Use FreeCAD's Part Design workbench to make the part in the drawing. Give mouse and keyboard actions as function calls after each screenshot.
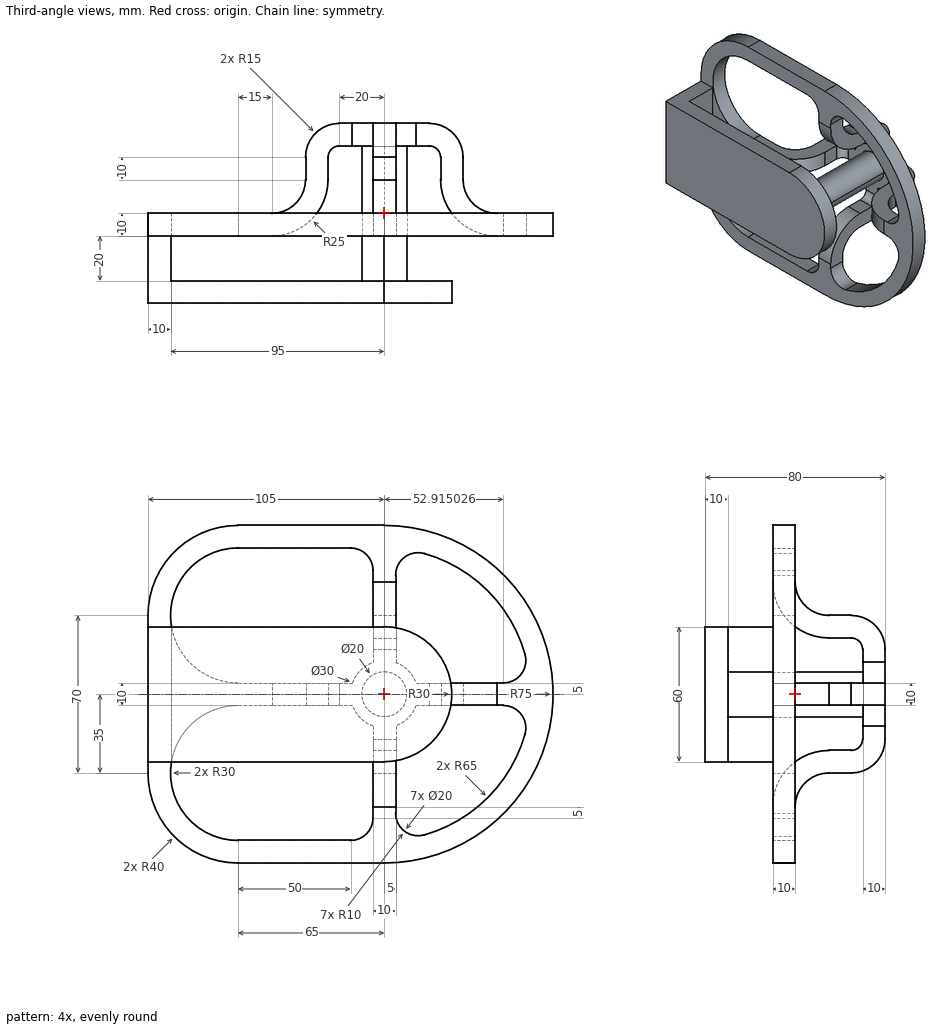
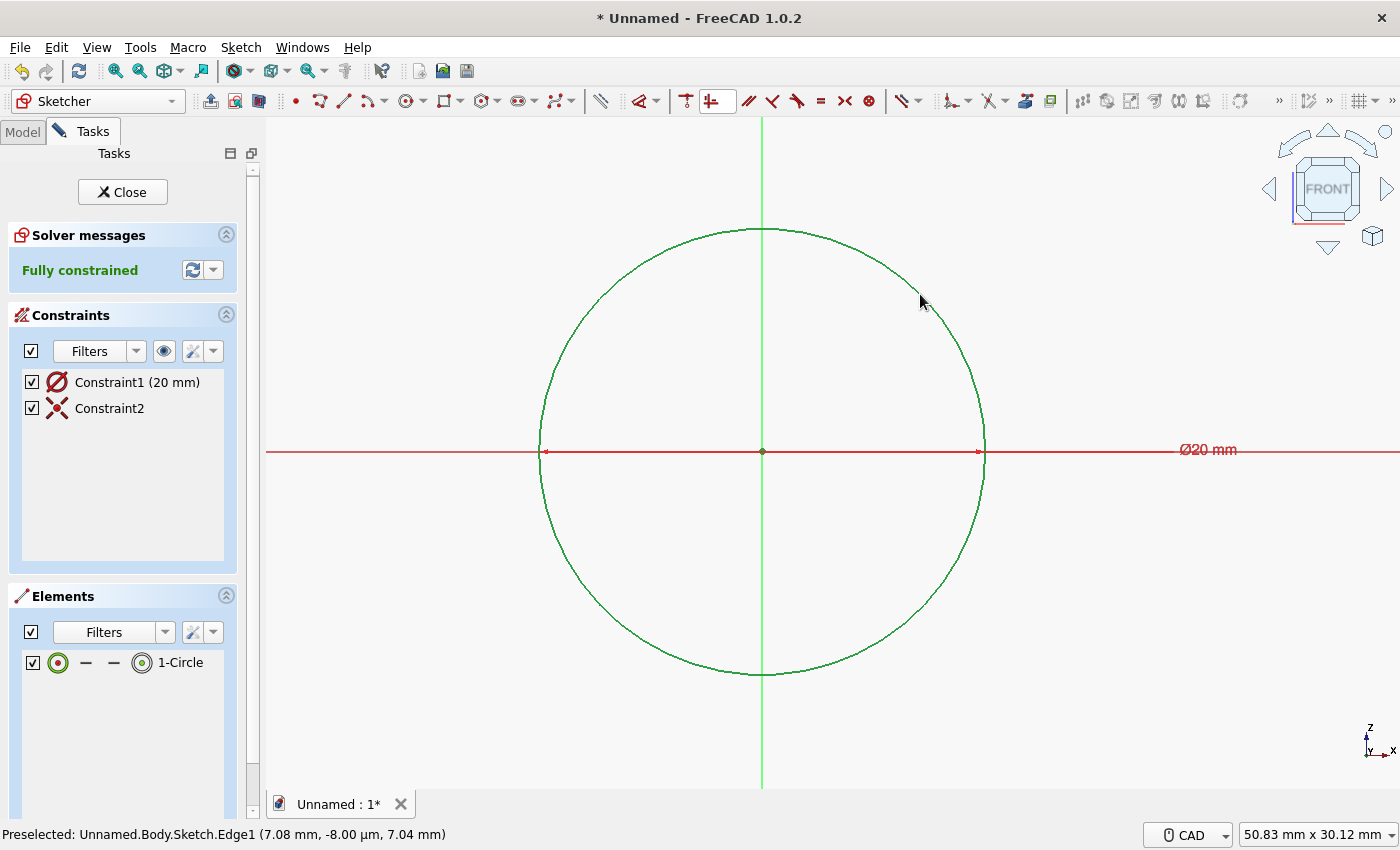
click(123, 192)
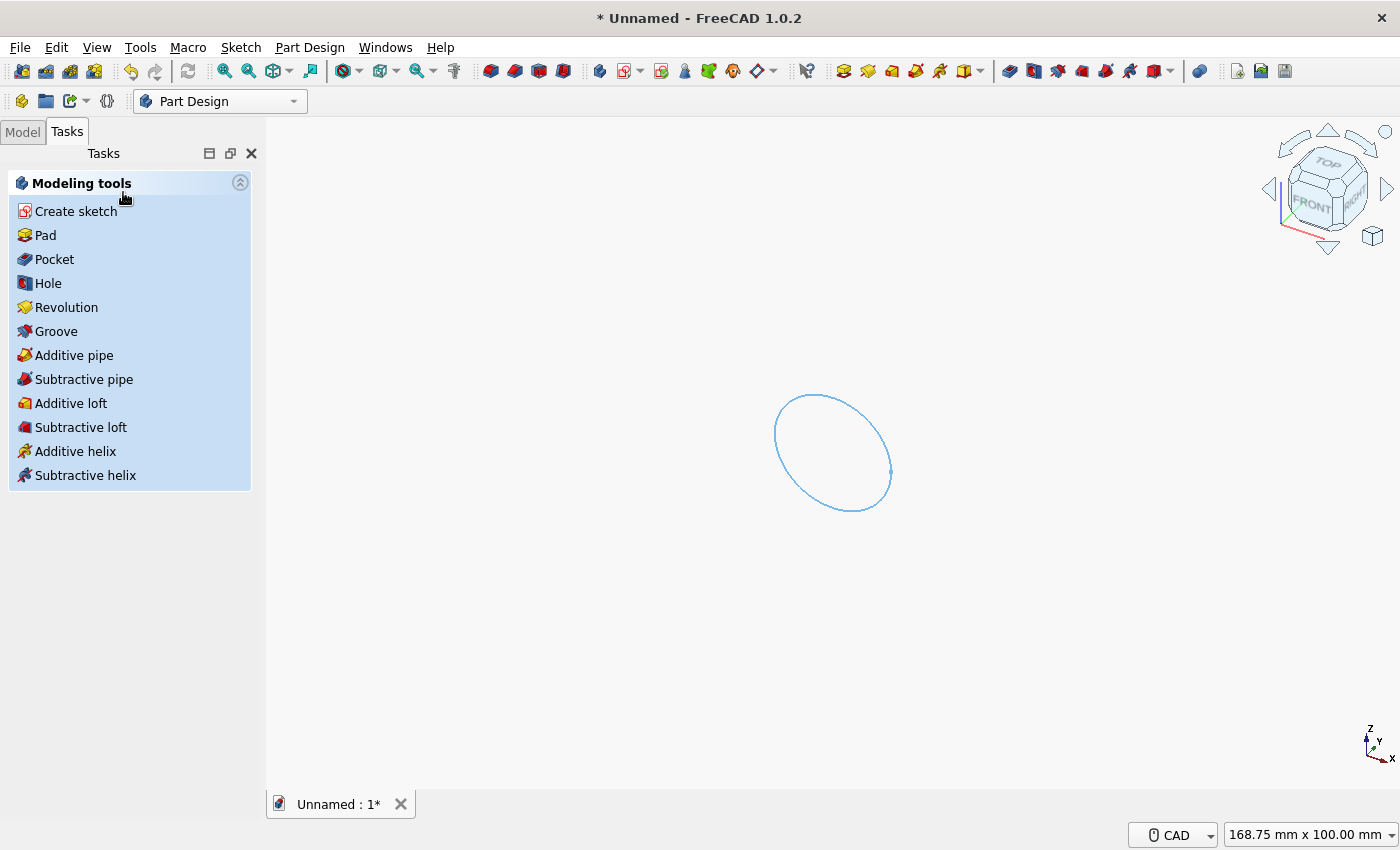
click(844, 72)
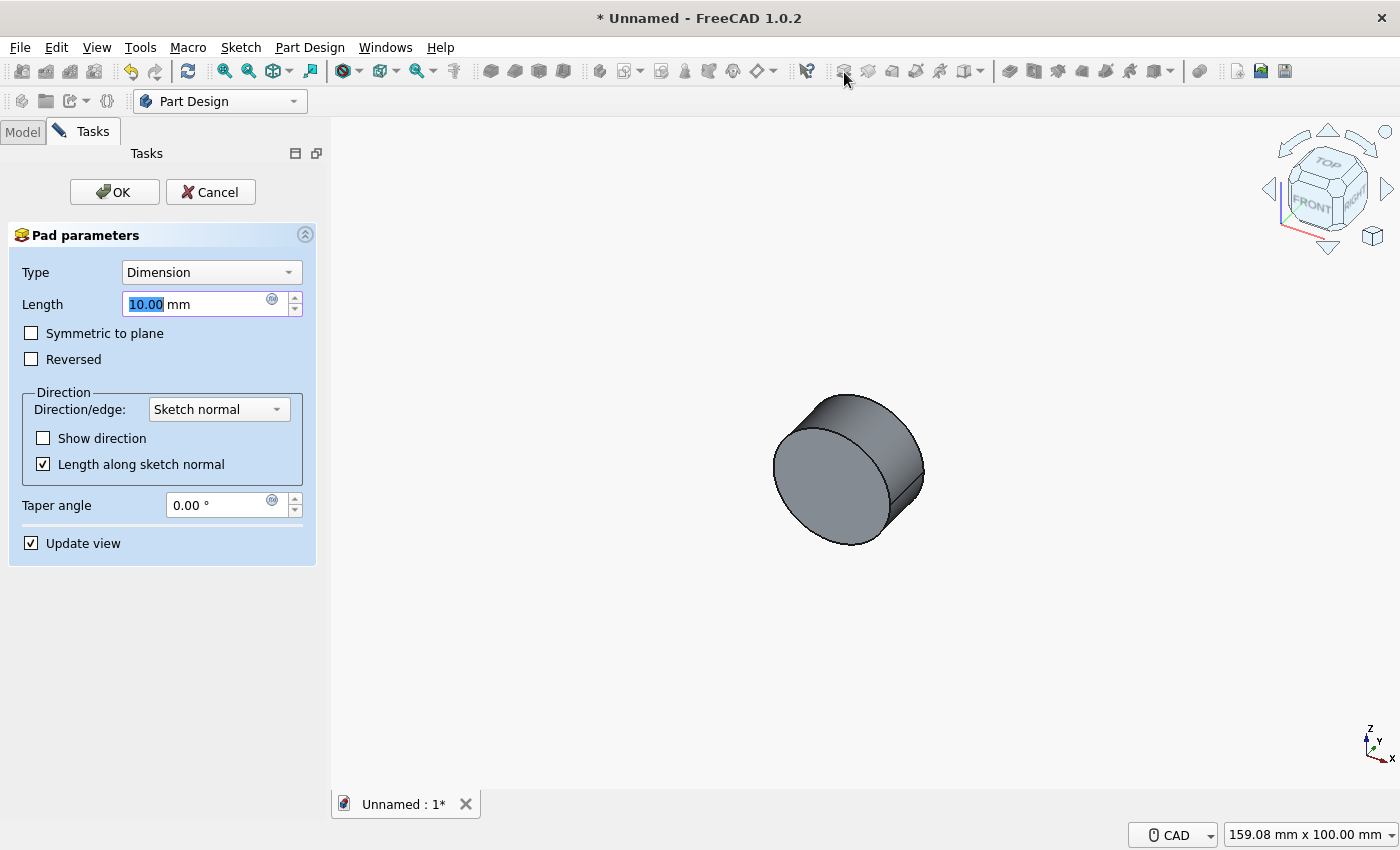
text(80)
key(Tab)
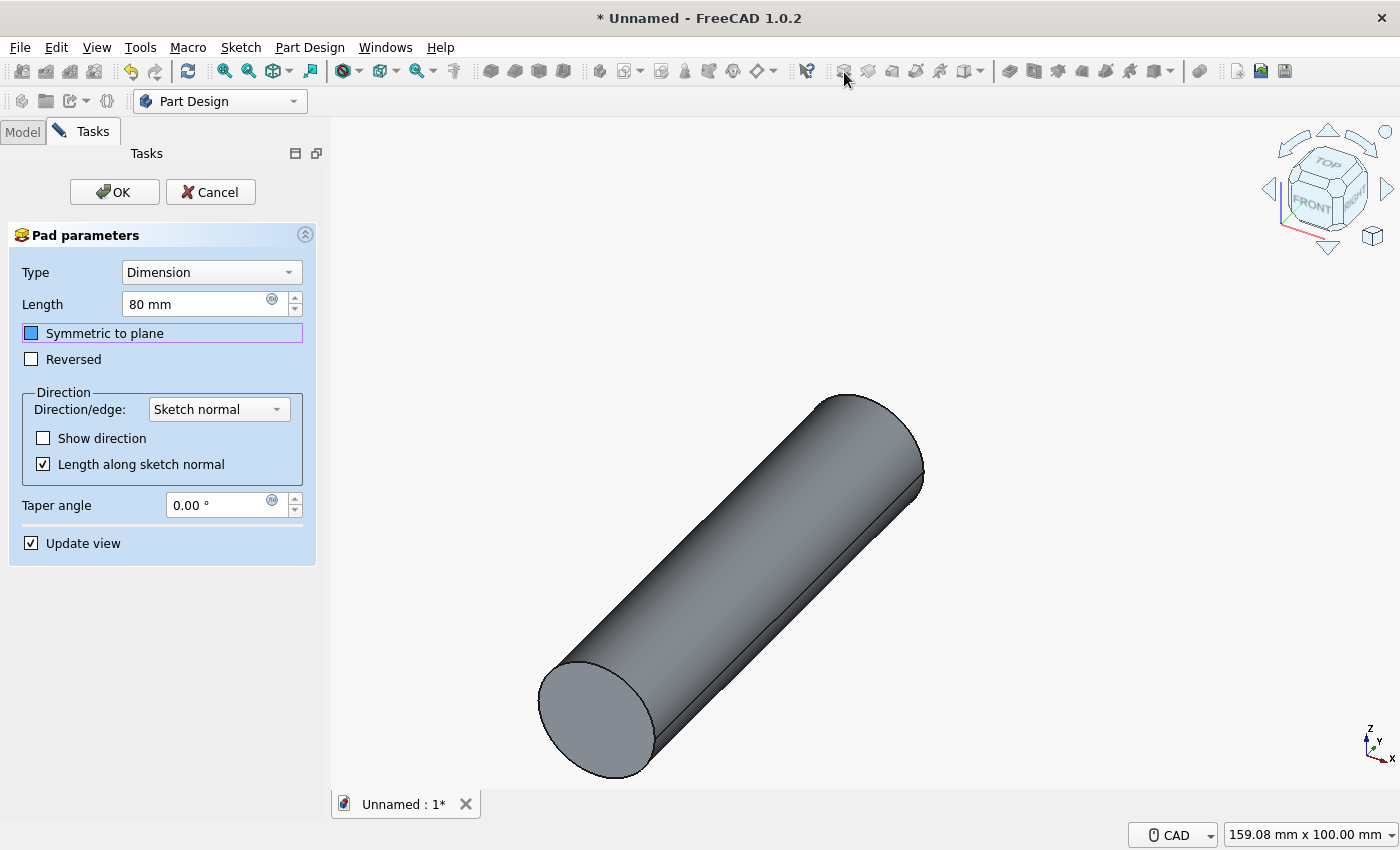
click(30, 333)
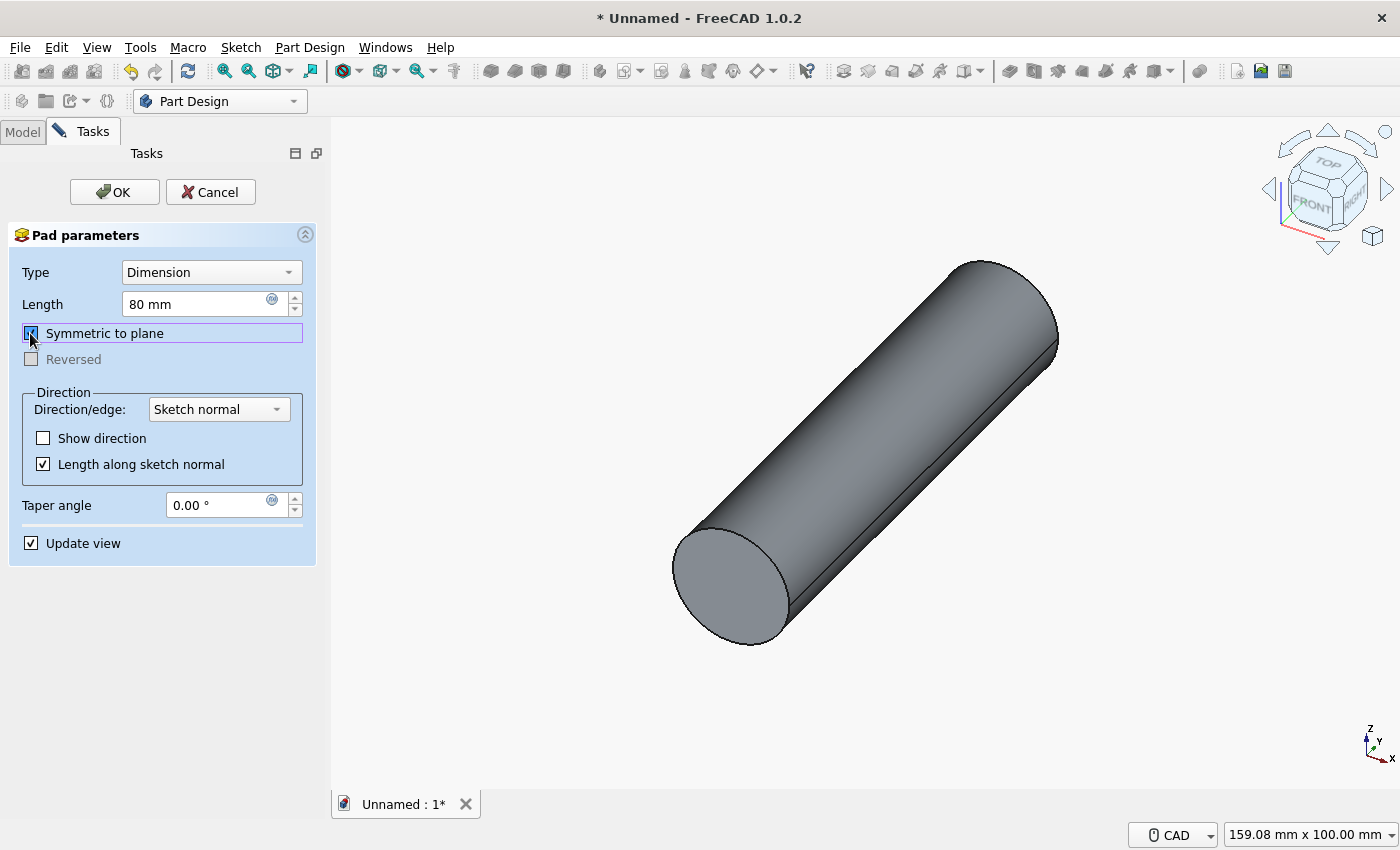
click(115, 192)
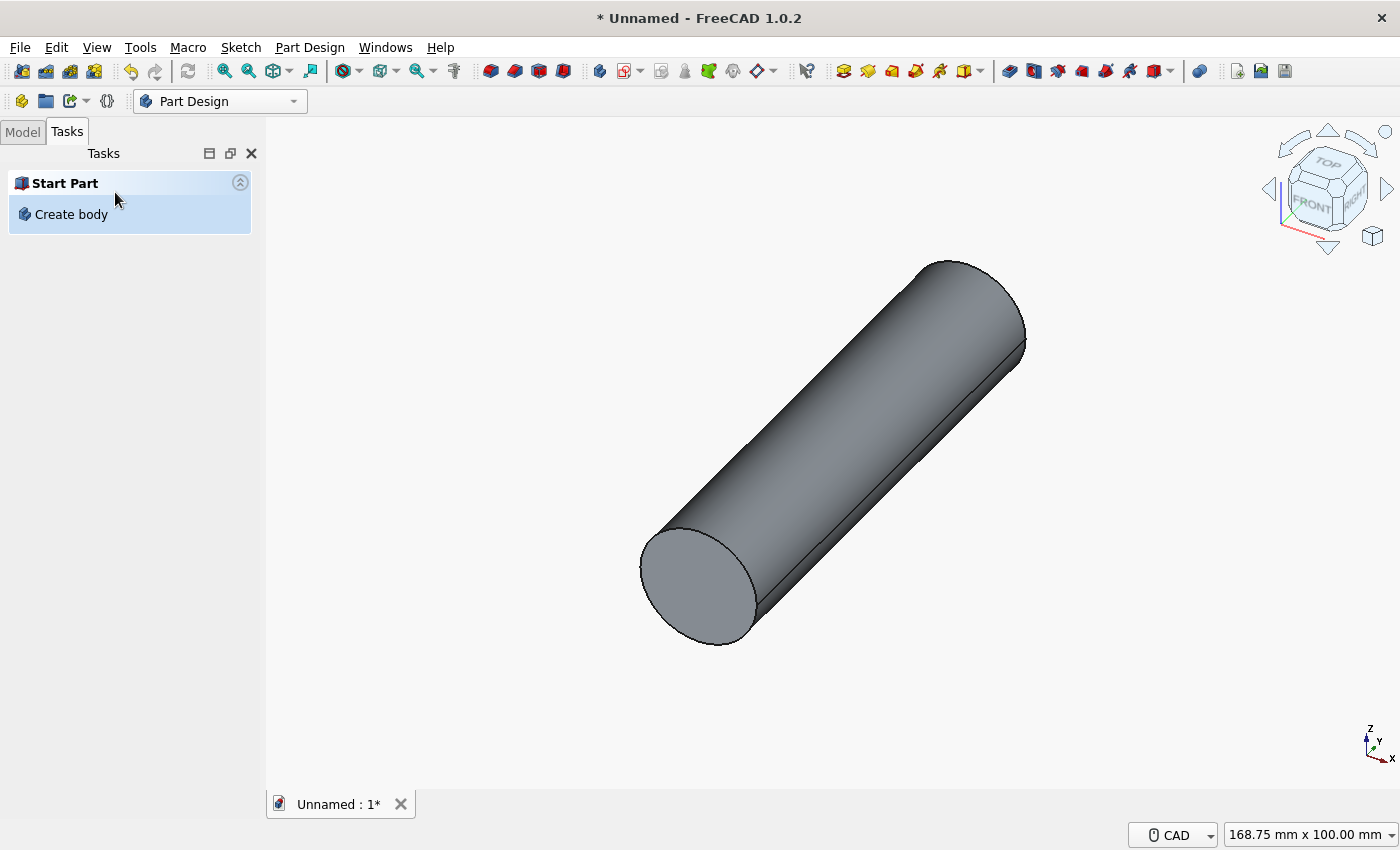
click(624, 72)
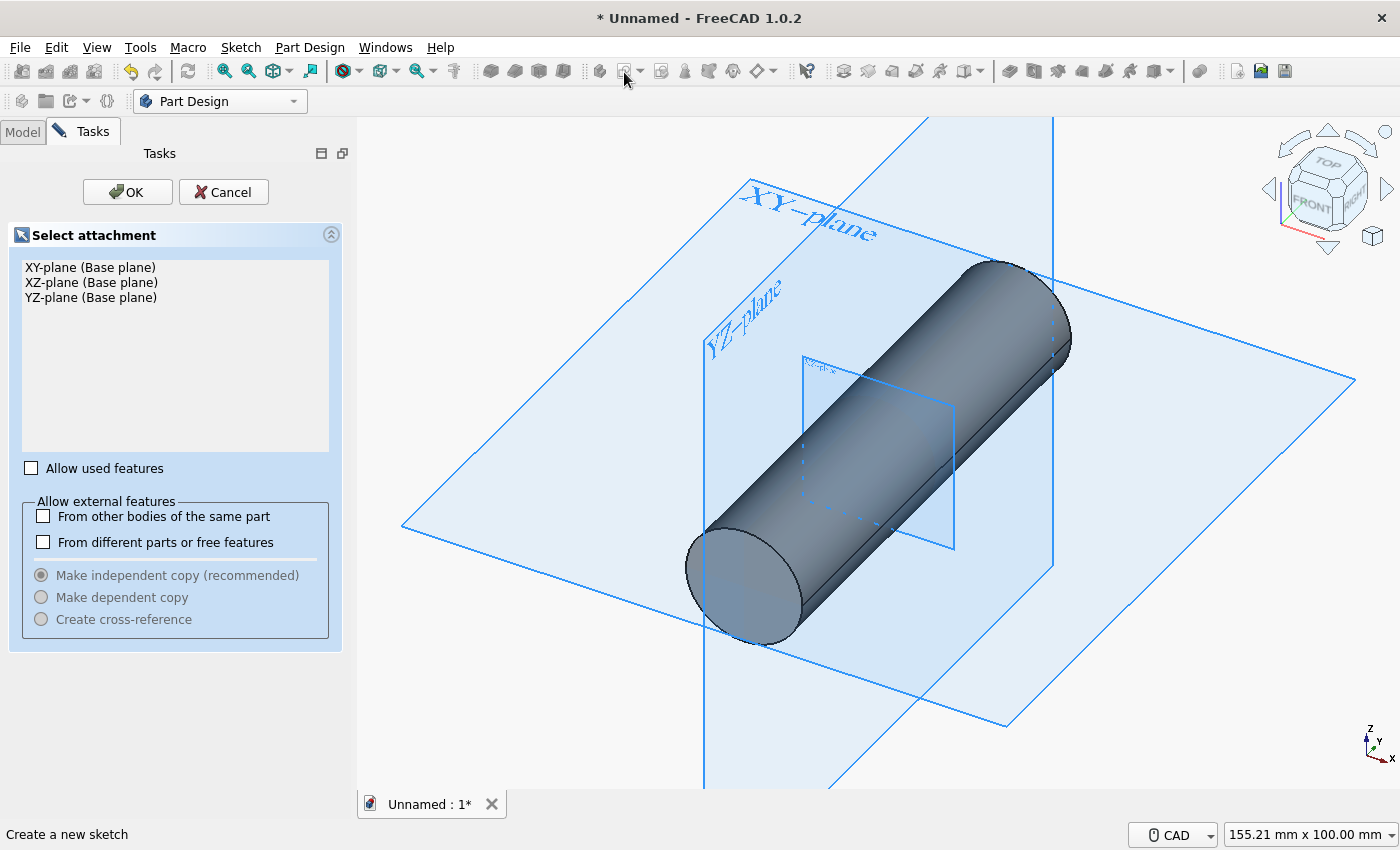
click(82, 282)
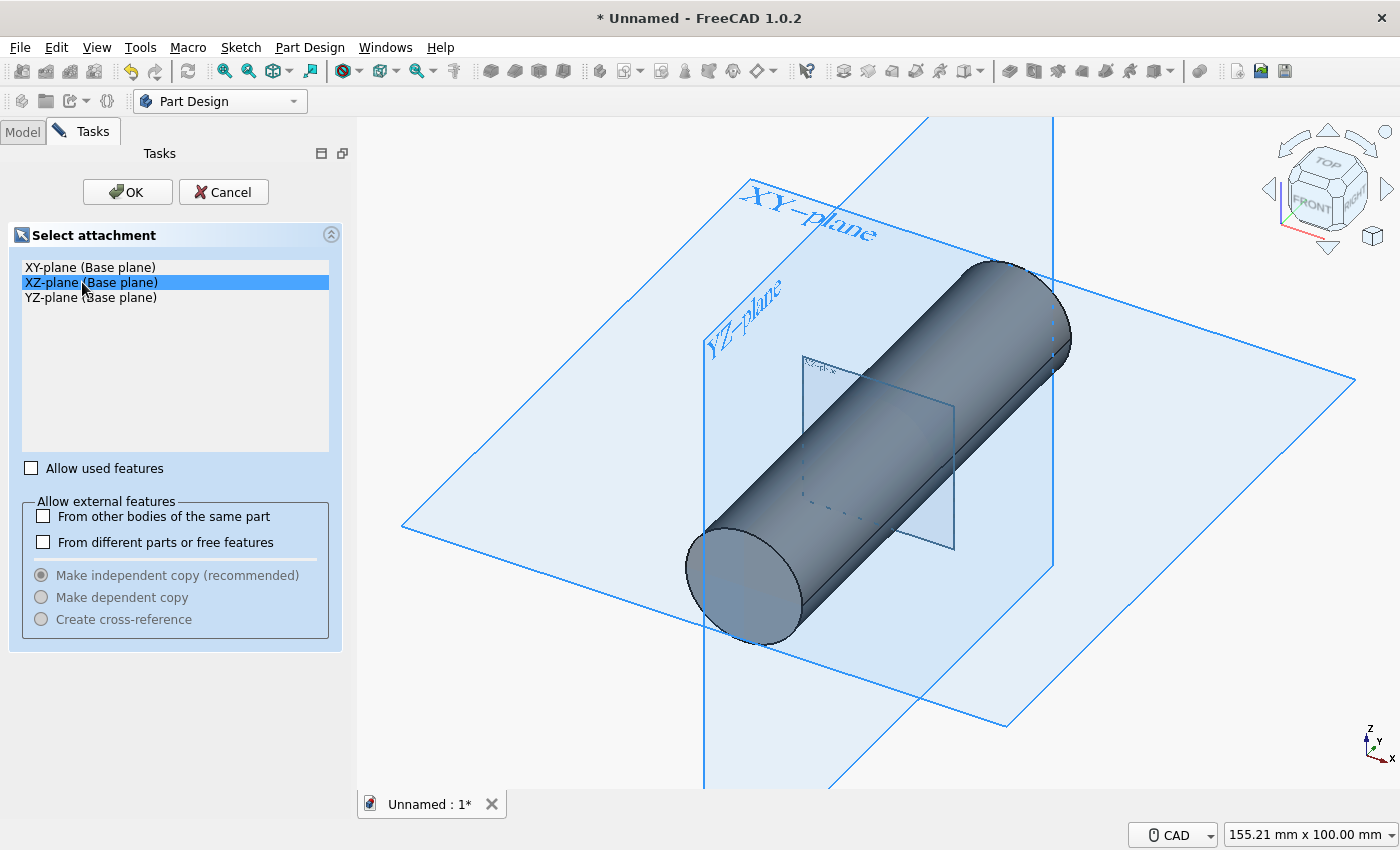
click(128, 192)